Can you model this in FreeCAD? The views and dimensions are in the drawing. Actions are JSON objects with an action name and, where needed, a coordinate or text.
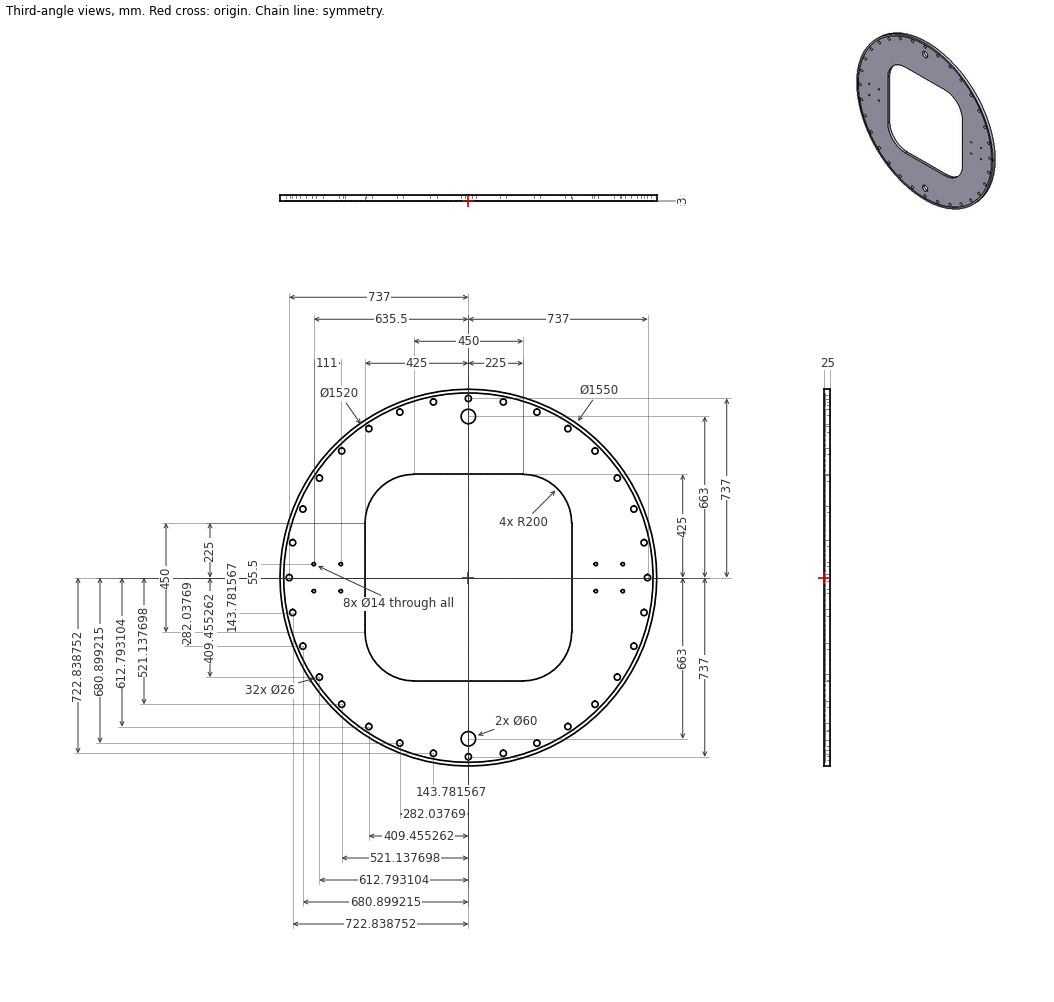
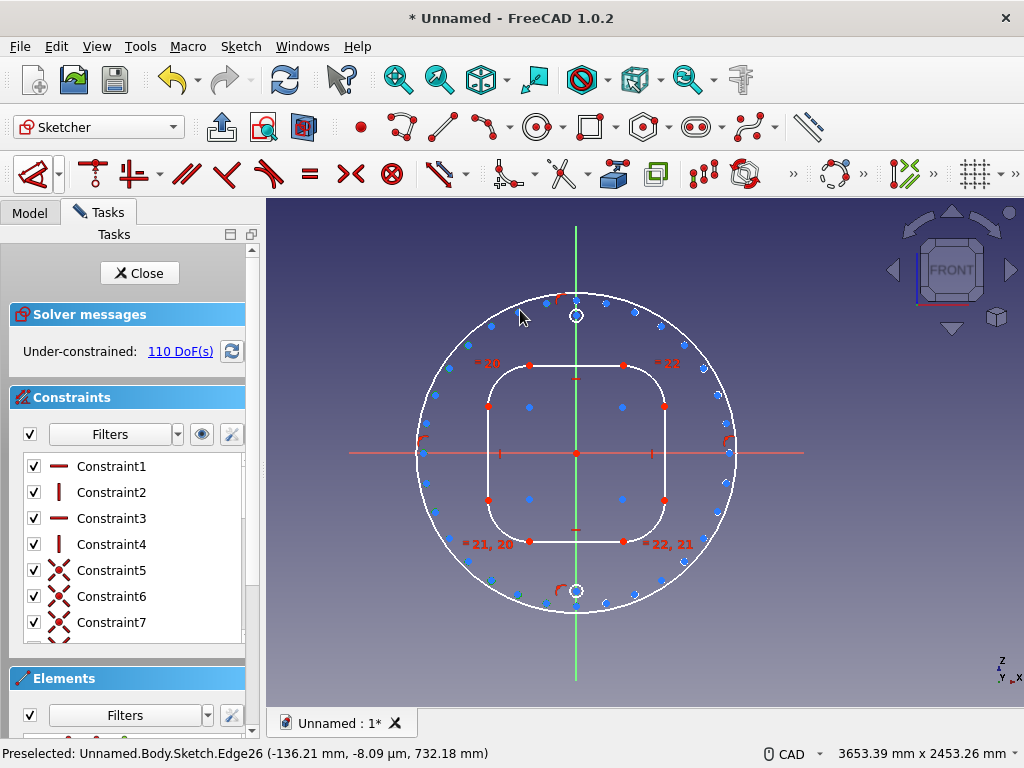
{"action": "scroll", "coordinate": [608, 601], "scroll_direction": "up", "scroll_amount": 8}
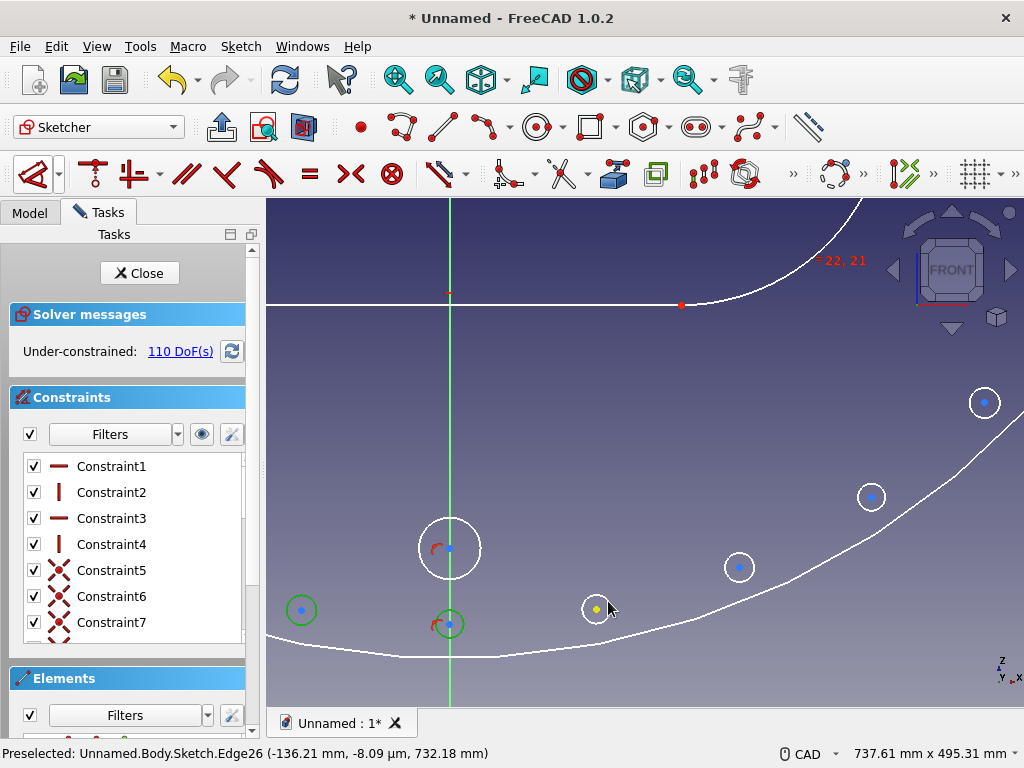
{"action": "left_click", "coordinate": [607, 599]}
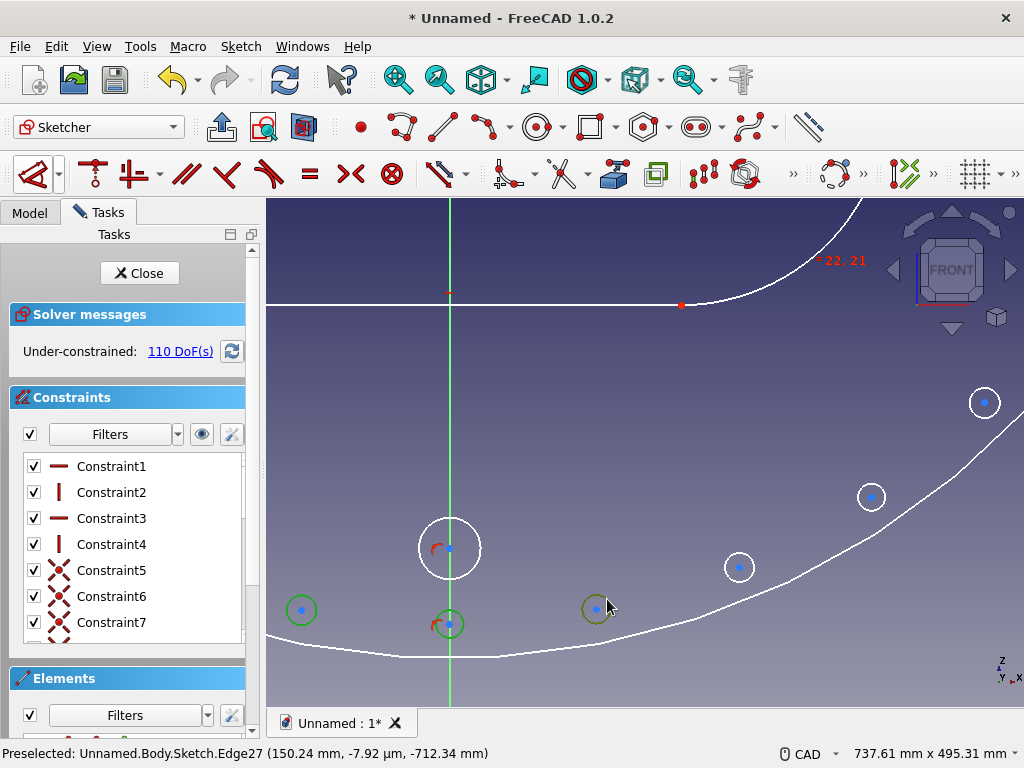
{"action": "left_click", "coordinate": [750, 557]}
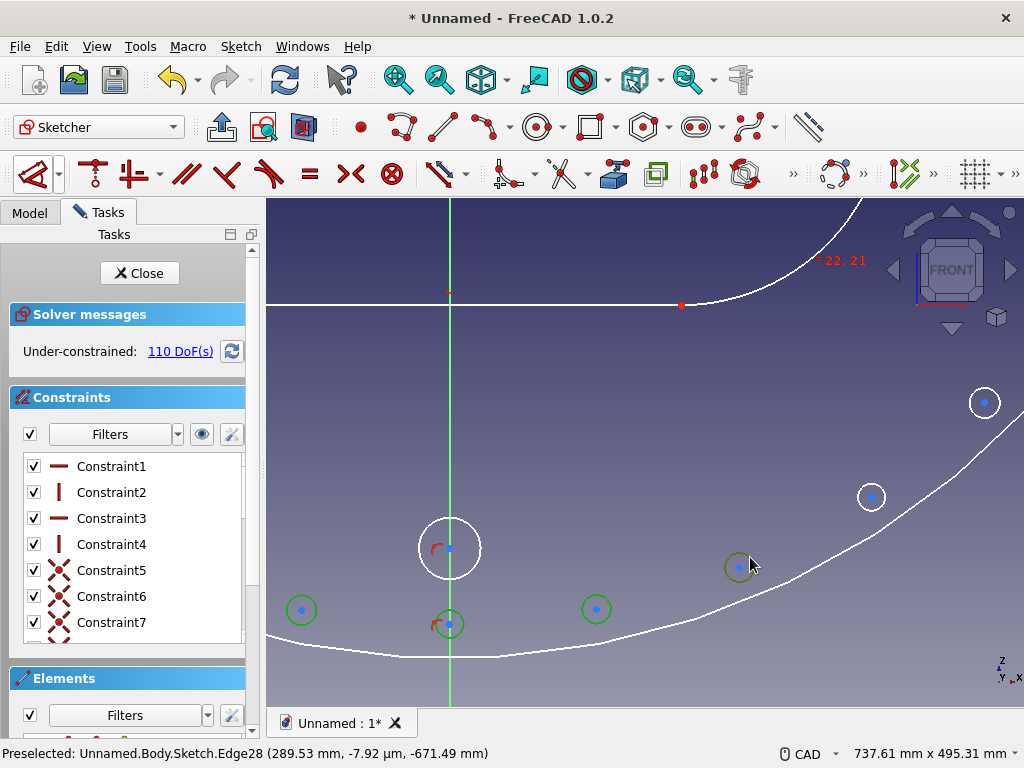
{"action": "left_click", "coordinate": [858, 497]}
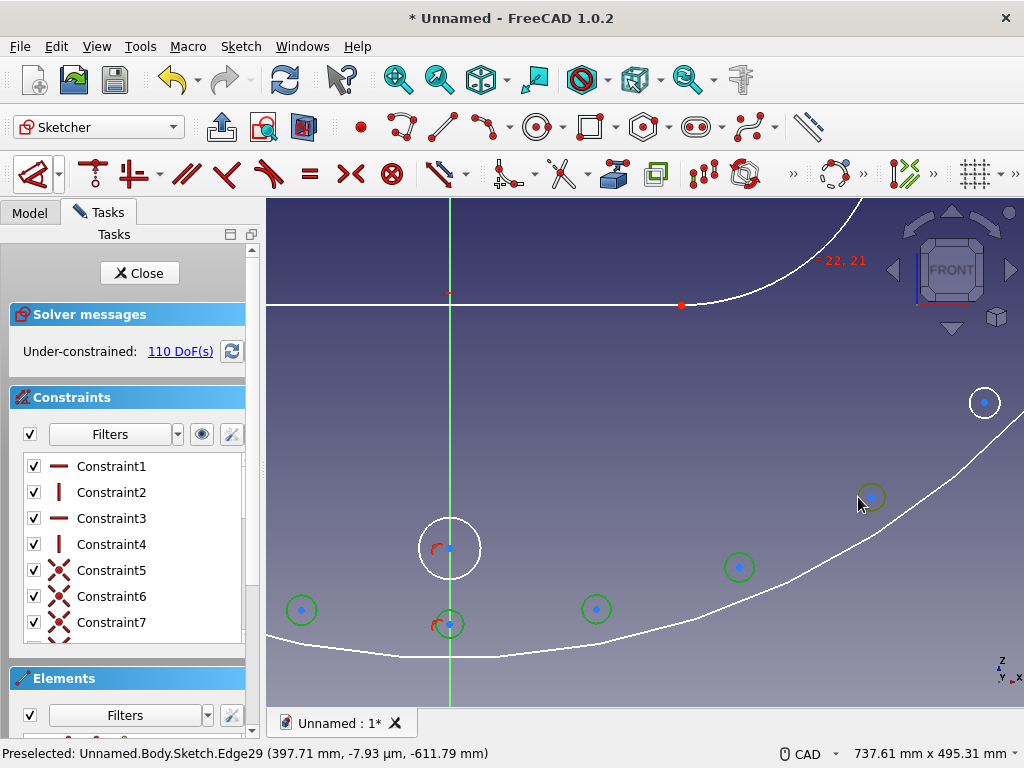
{"action": "scroll", "coordinate": [609, 601], "scroll_direction": "down", "scroll_amount": 8}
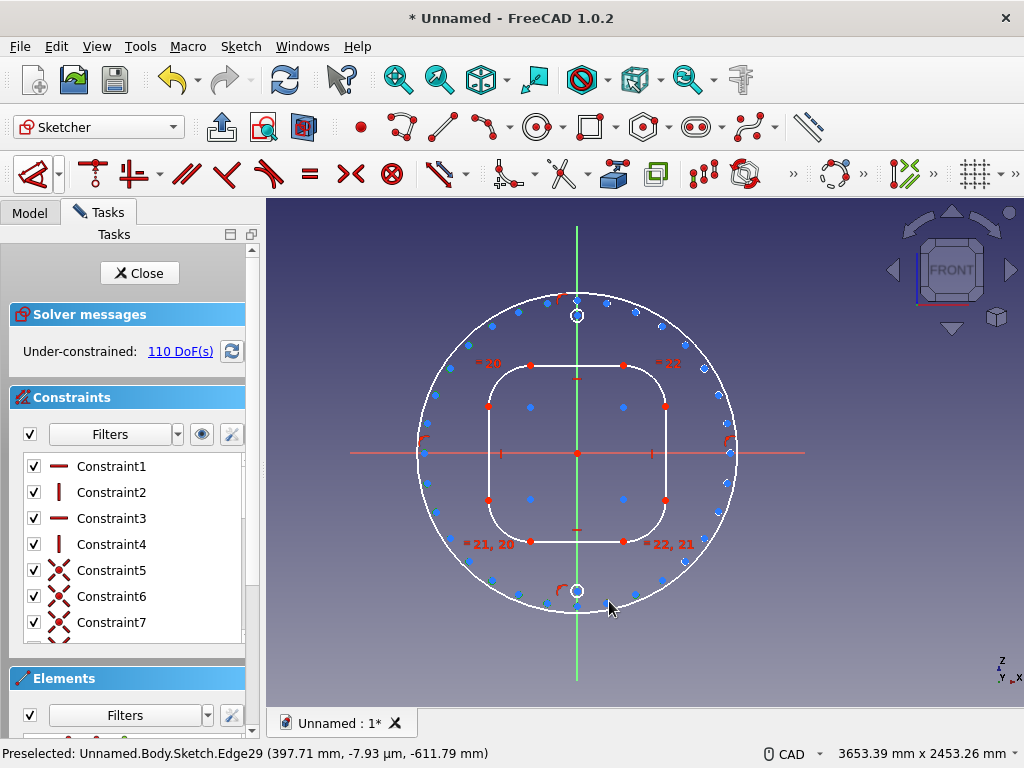
{"action": "scroll", "coordinate": [687, 560], "scroll_direction": "up", "scroll_amount": 8}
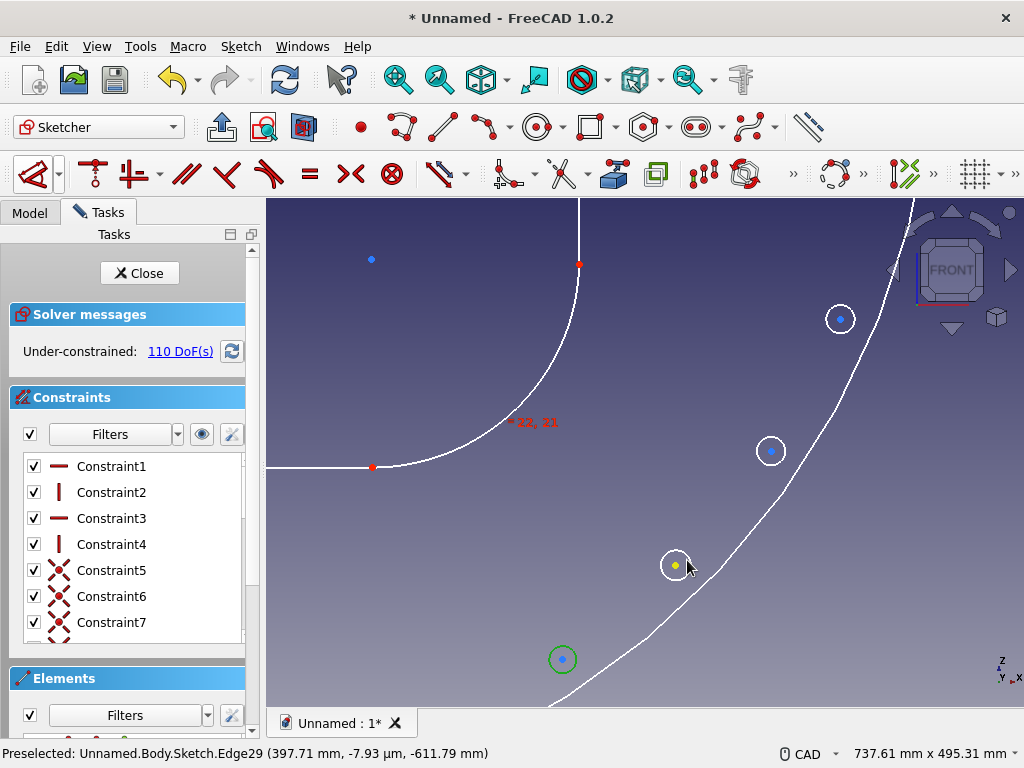
{"action": "left_click", "coordinate": [687, 555]}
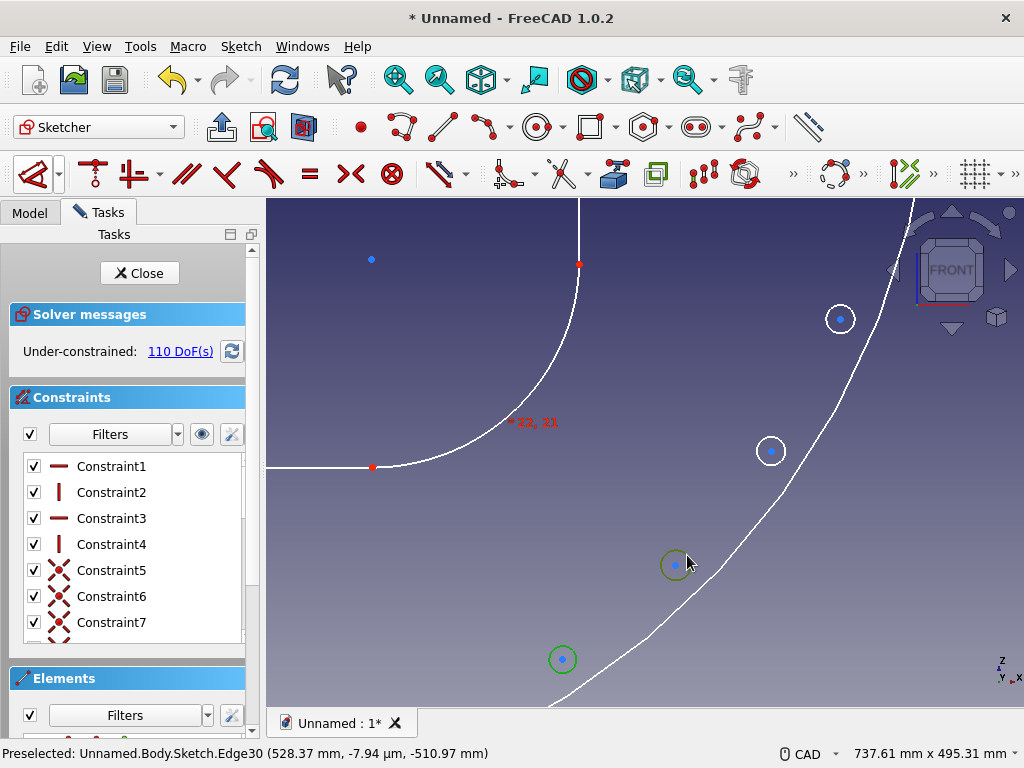
{"action": "left_click", "coordinate": [781, 441]}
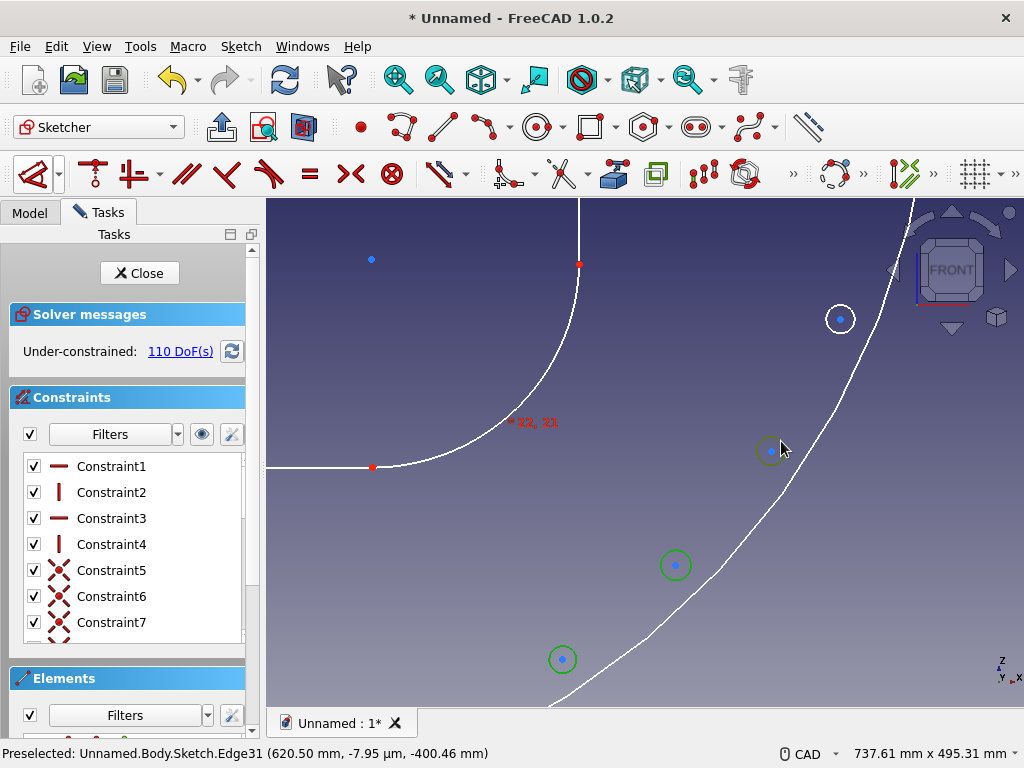
{"action": "left_click", "coordinate": [850, 309]}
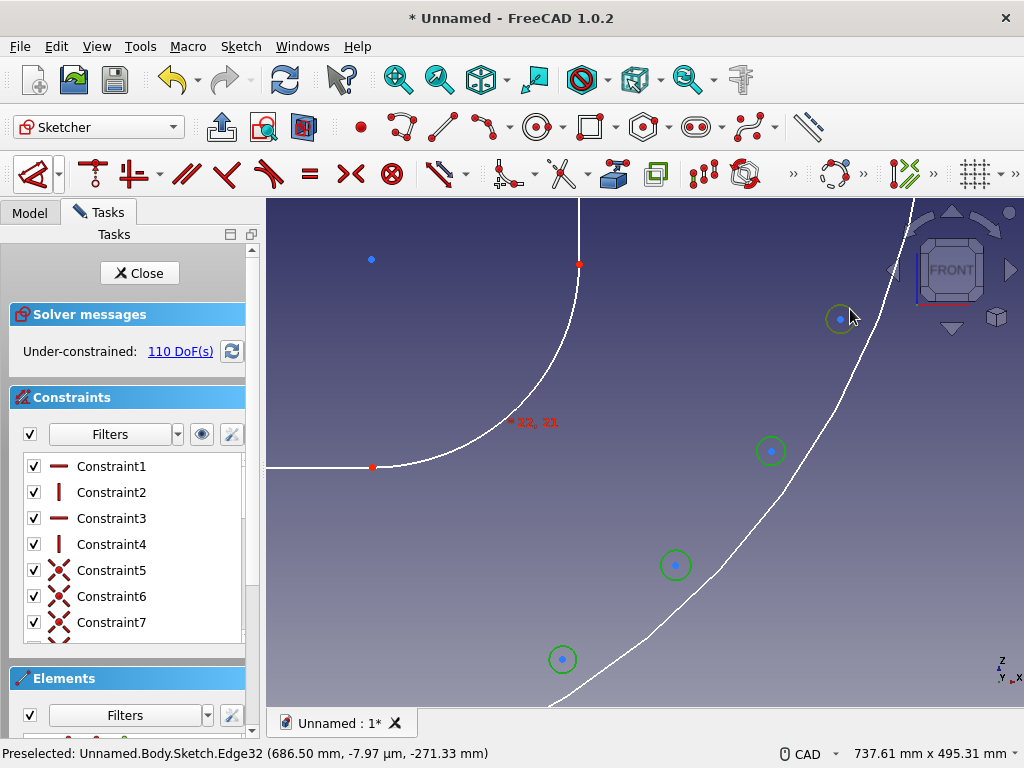
{"action": "scroll", "coordinate": [687, 560], "scroll_direction": "down", "scroll_amount": 8}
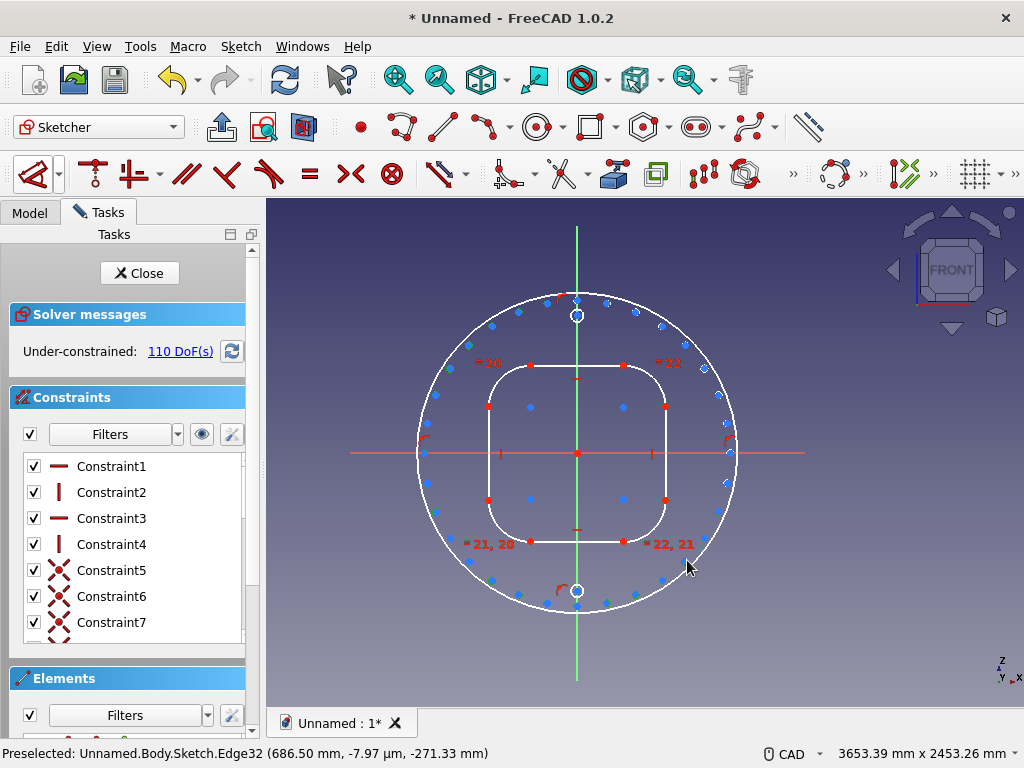
{"action": "scroll", "coordinate": [729, 481], "scroll_direction": "up", "scroll_amount": 8}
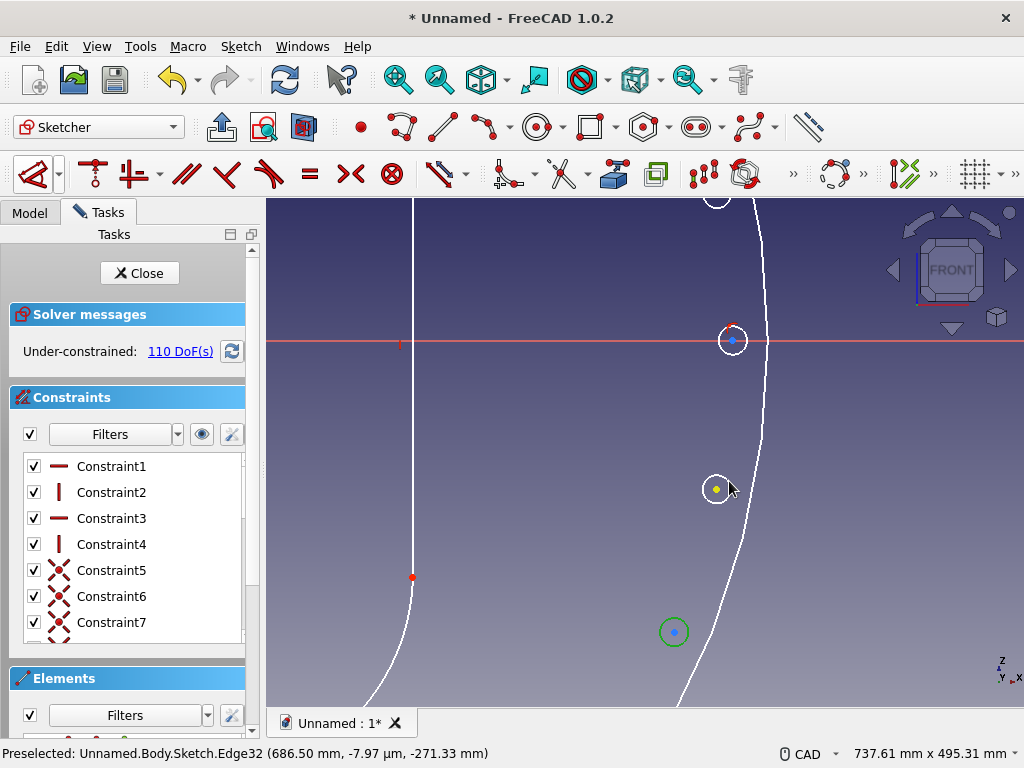
{"action": "left_click", "coordinate": [727, 479]}